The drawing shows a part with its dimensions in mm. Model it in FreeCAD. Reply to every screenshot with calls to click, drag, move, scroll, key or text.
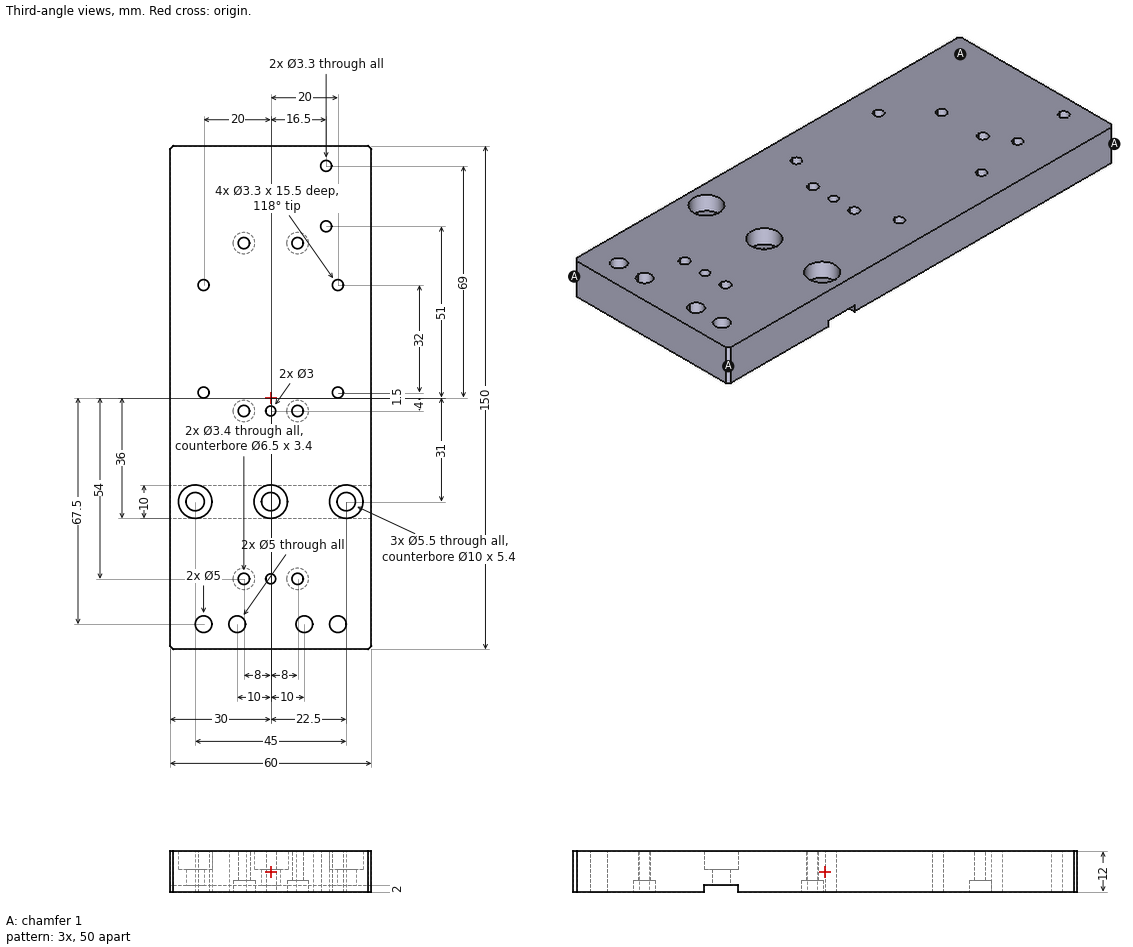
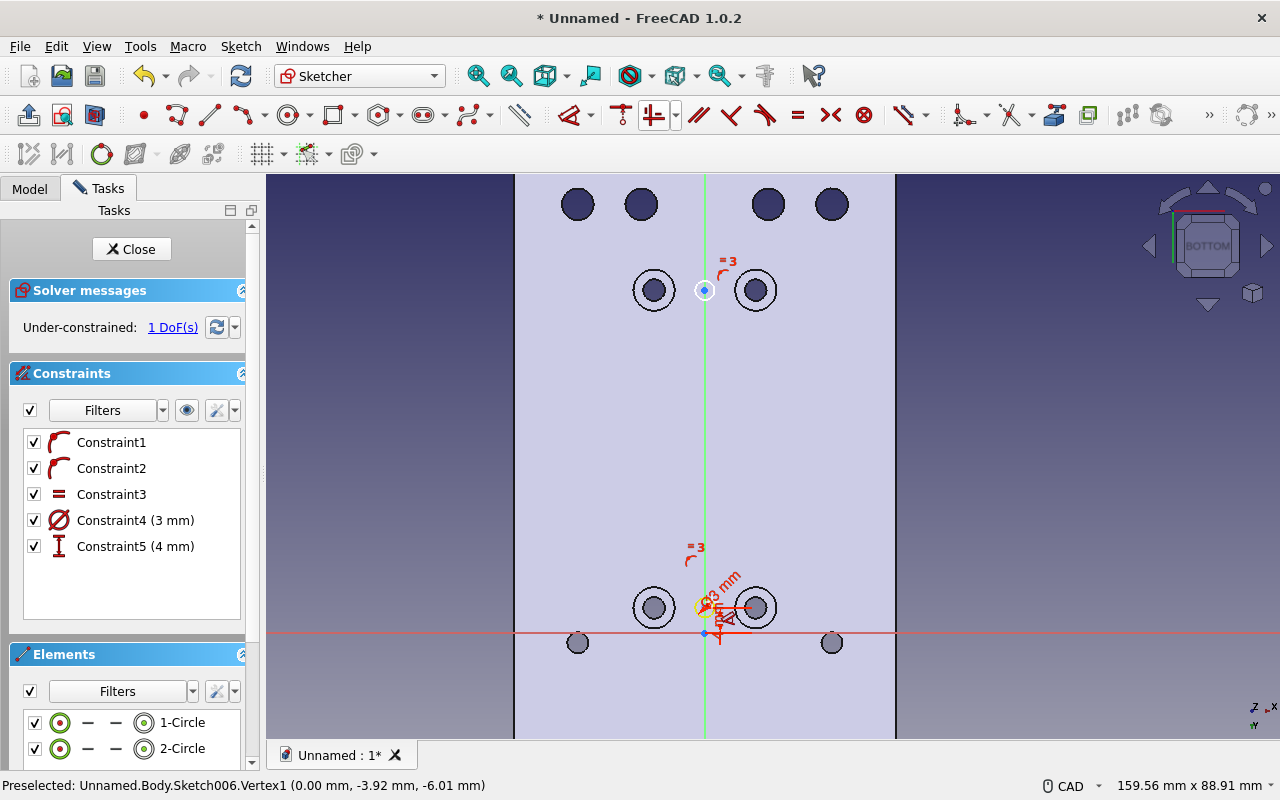
click(705, 290)
click(739, 462)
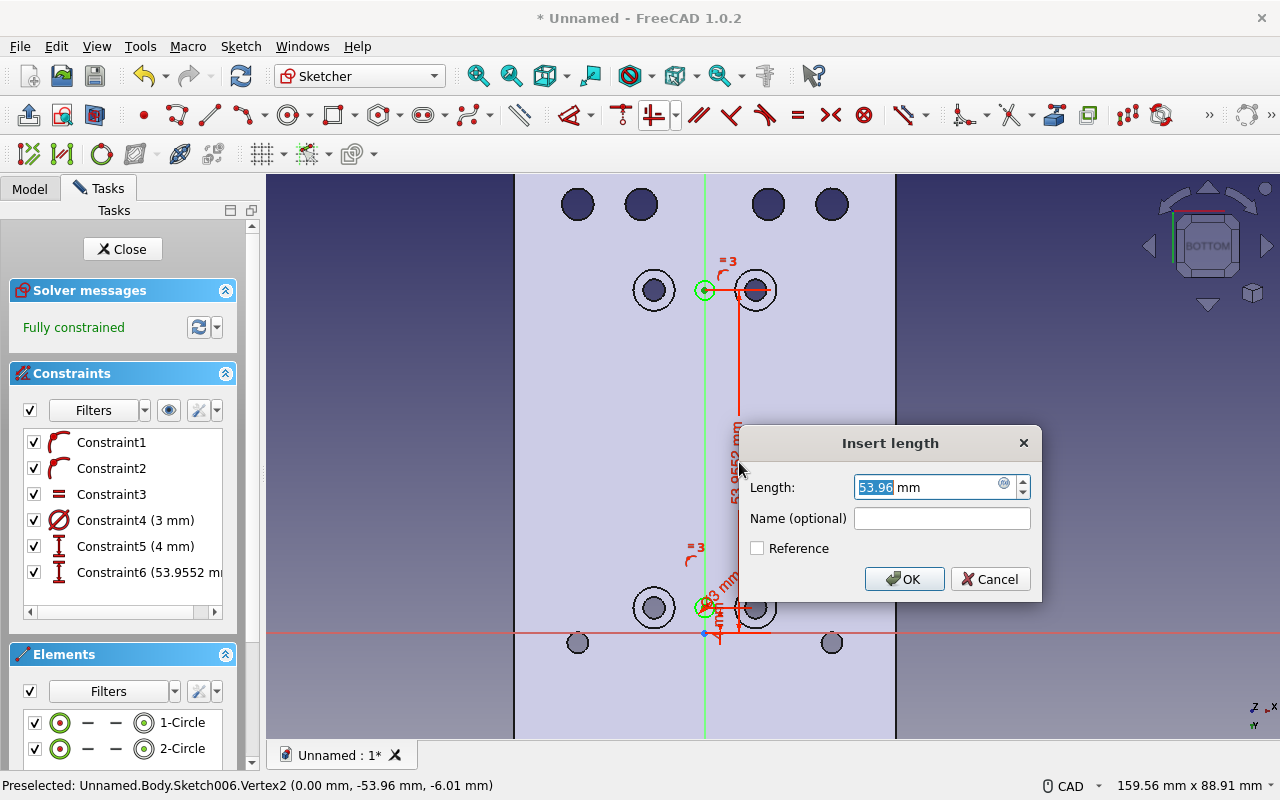
text(54)
key(Return)
key(Escape)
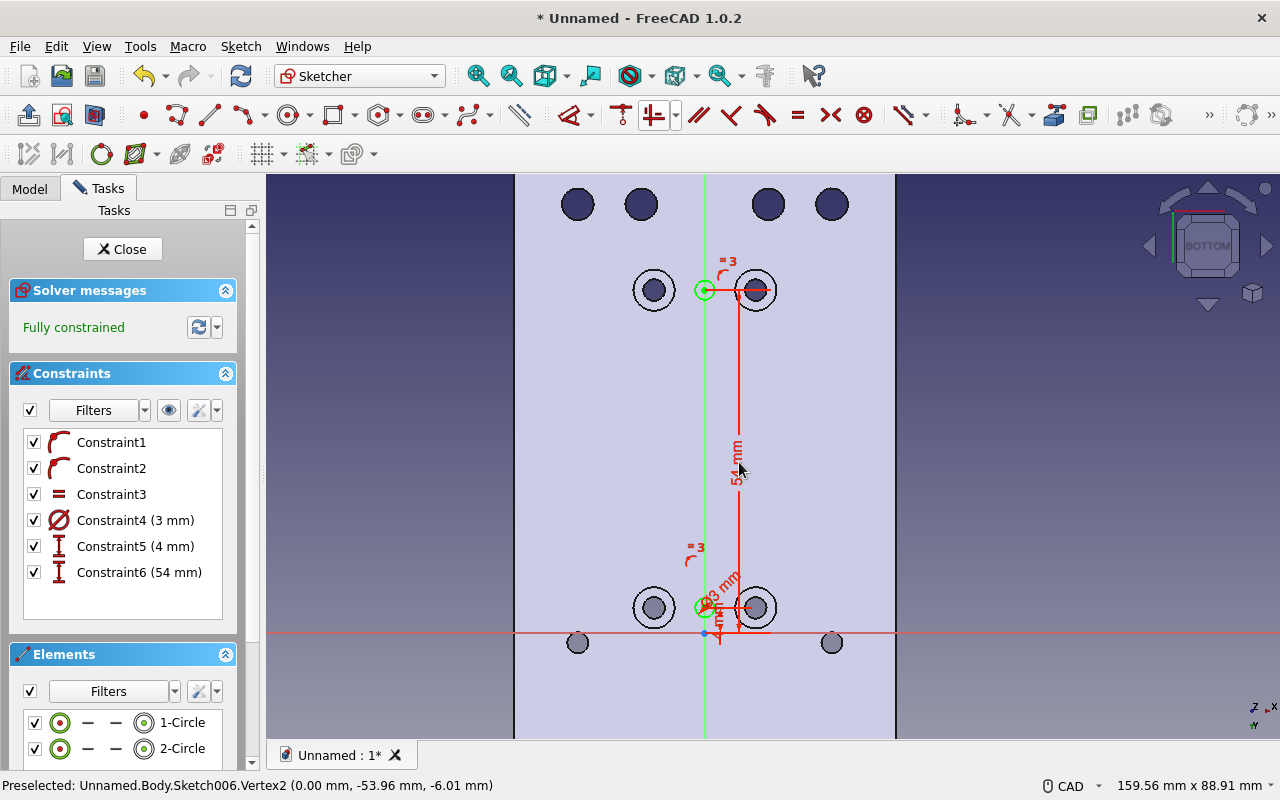
click(123, 249)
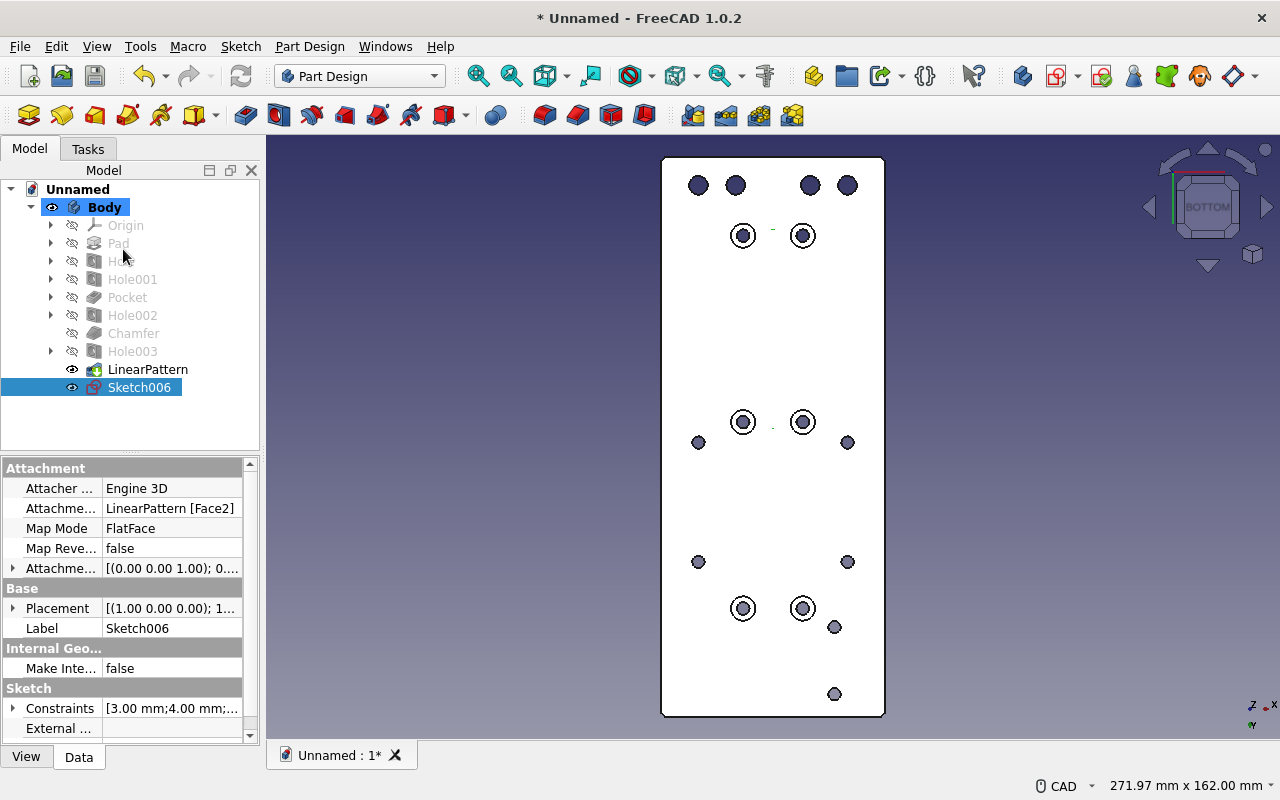
click(246, 116)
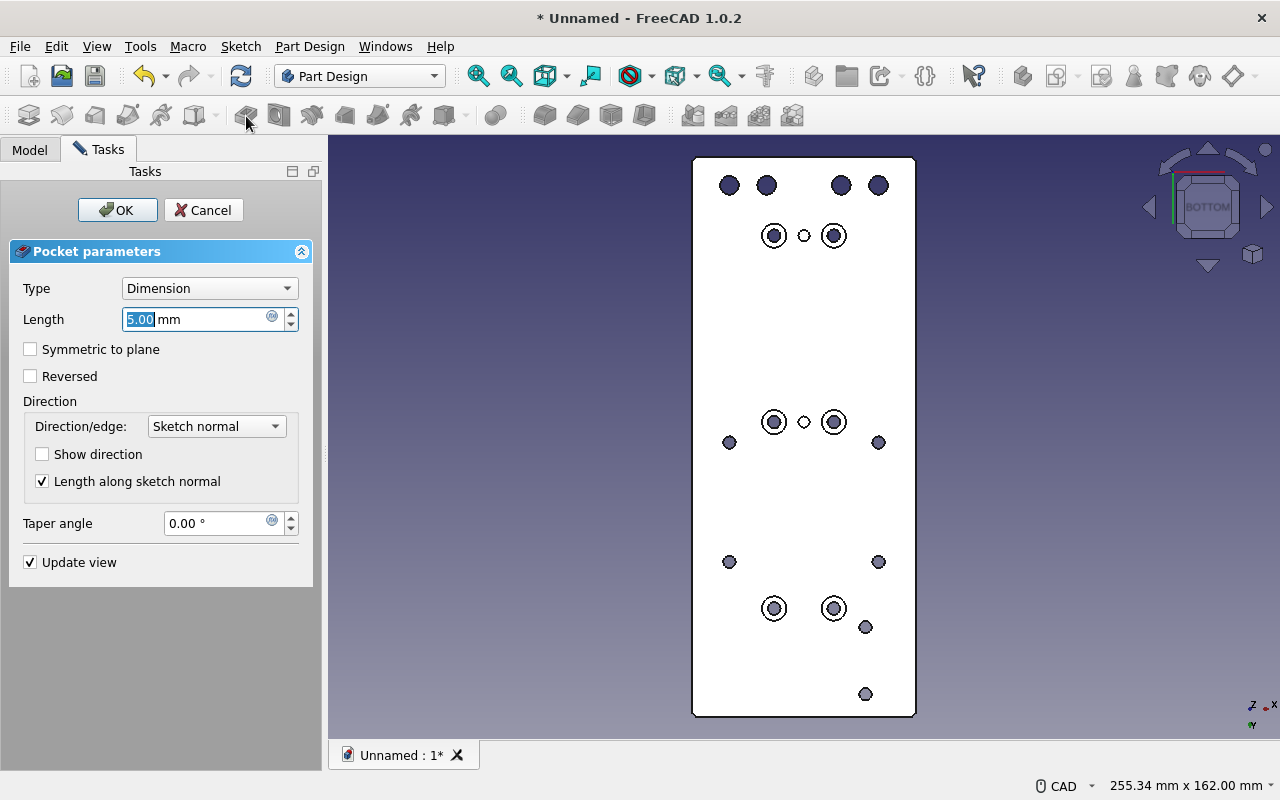
click(210, 288)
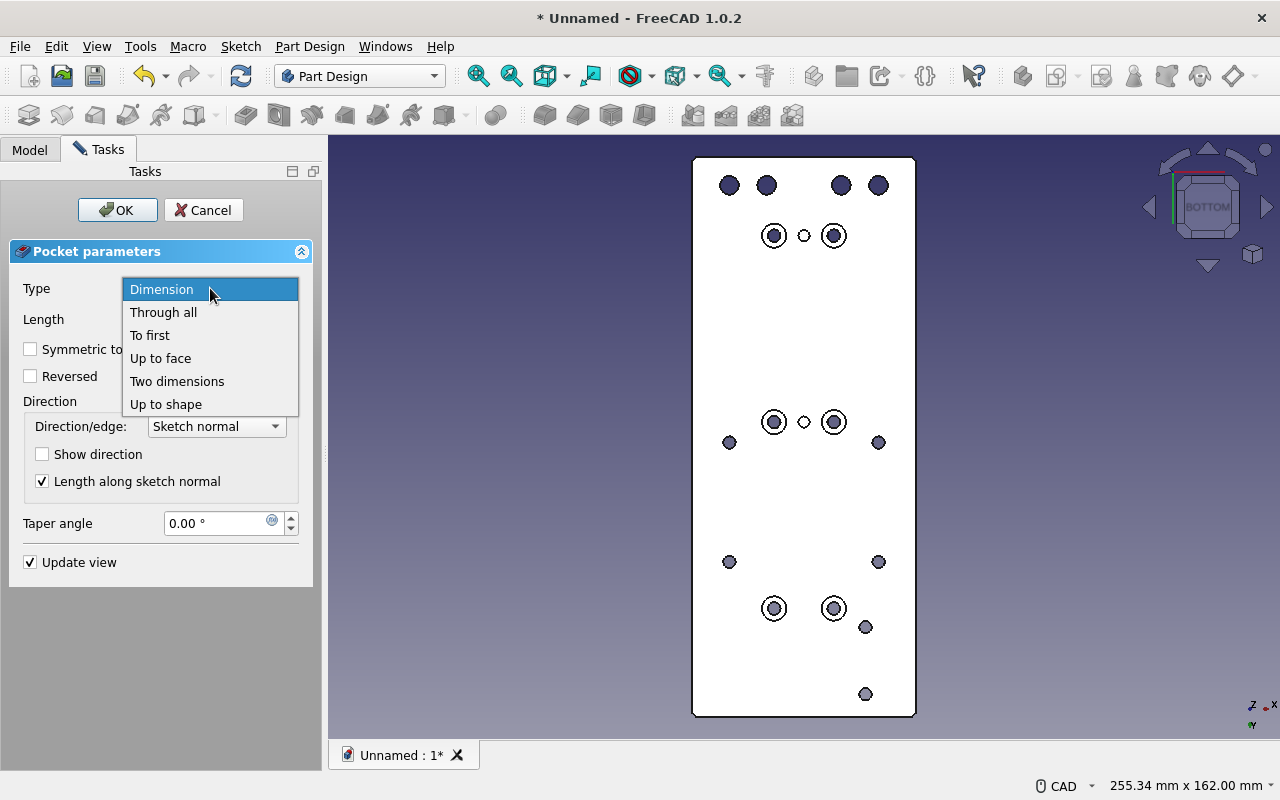
click(208, 312)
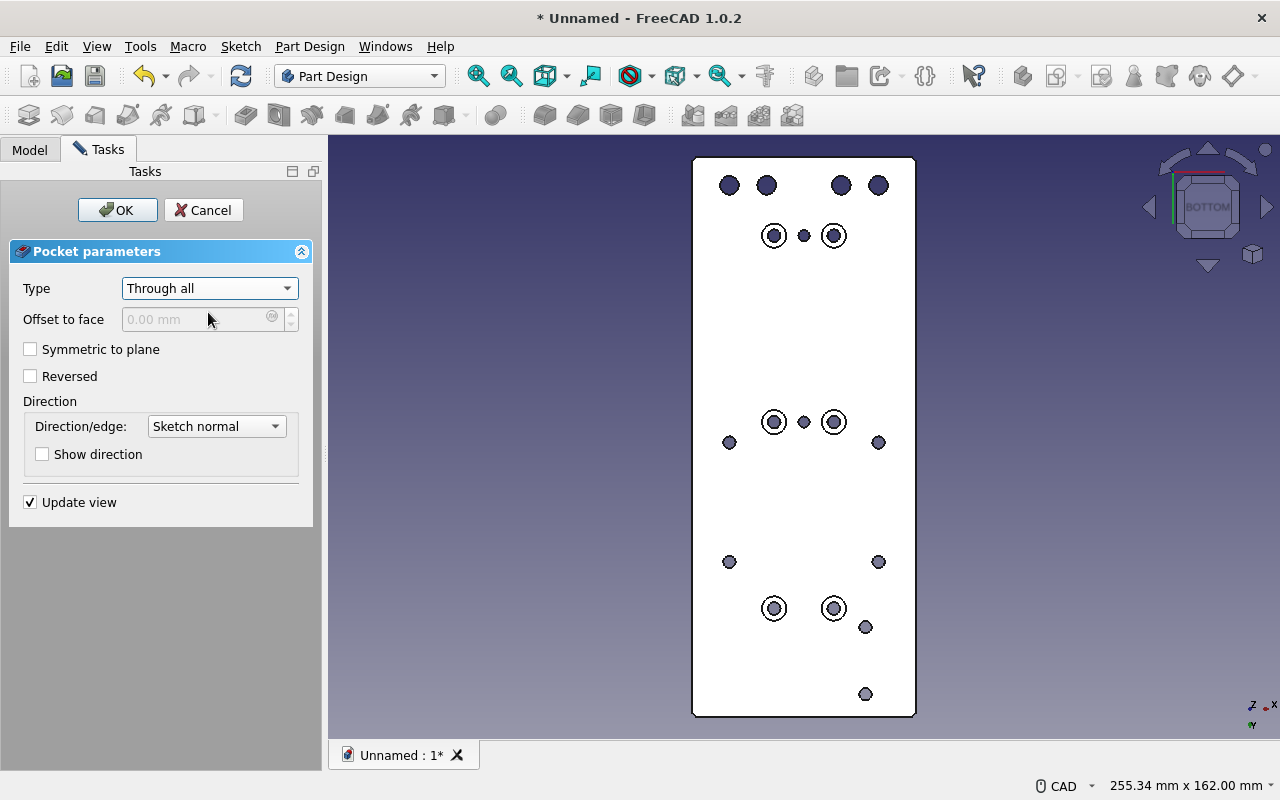
click(118, 210)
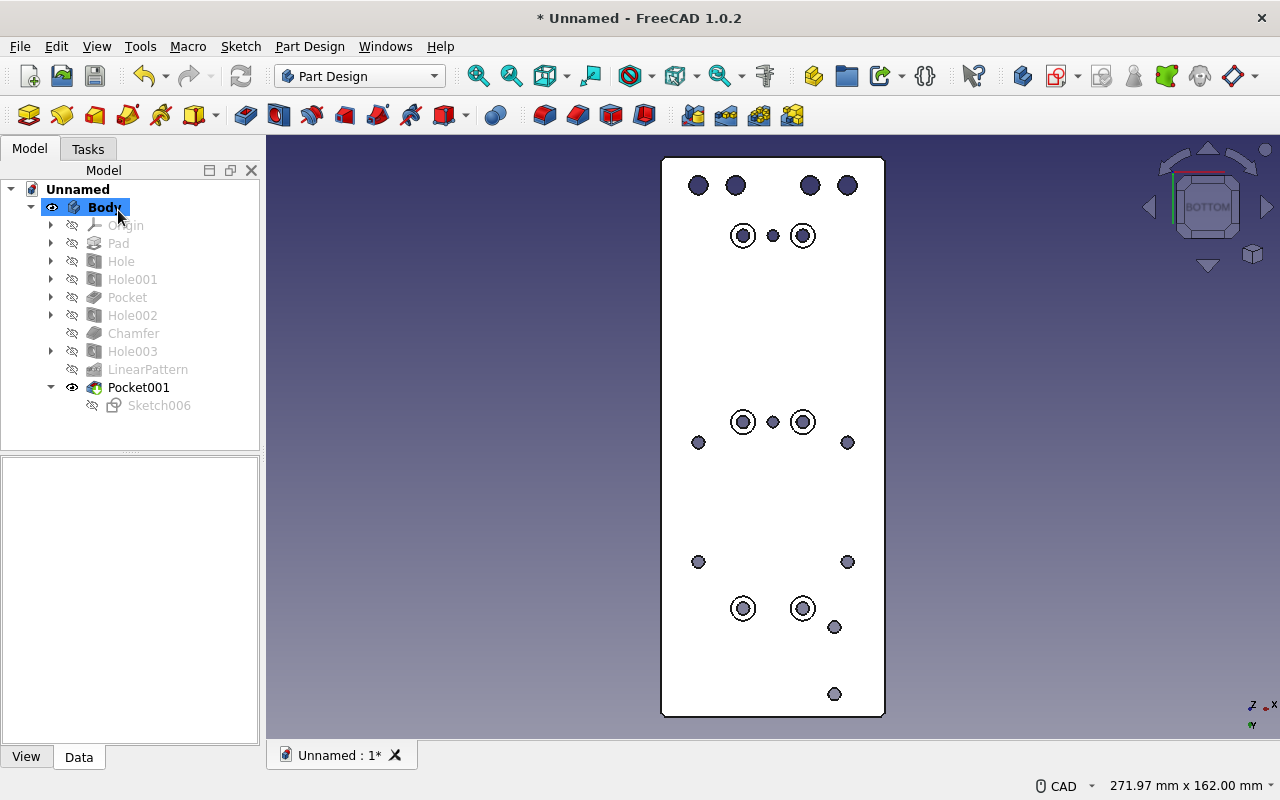
click(773, 516)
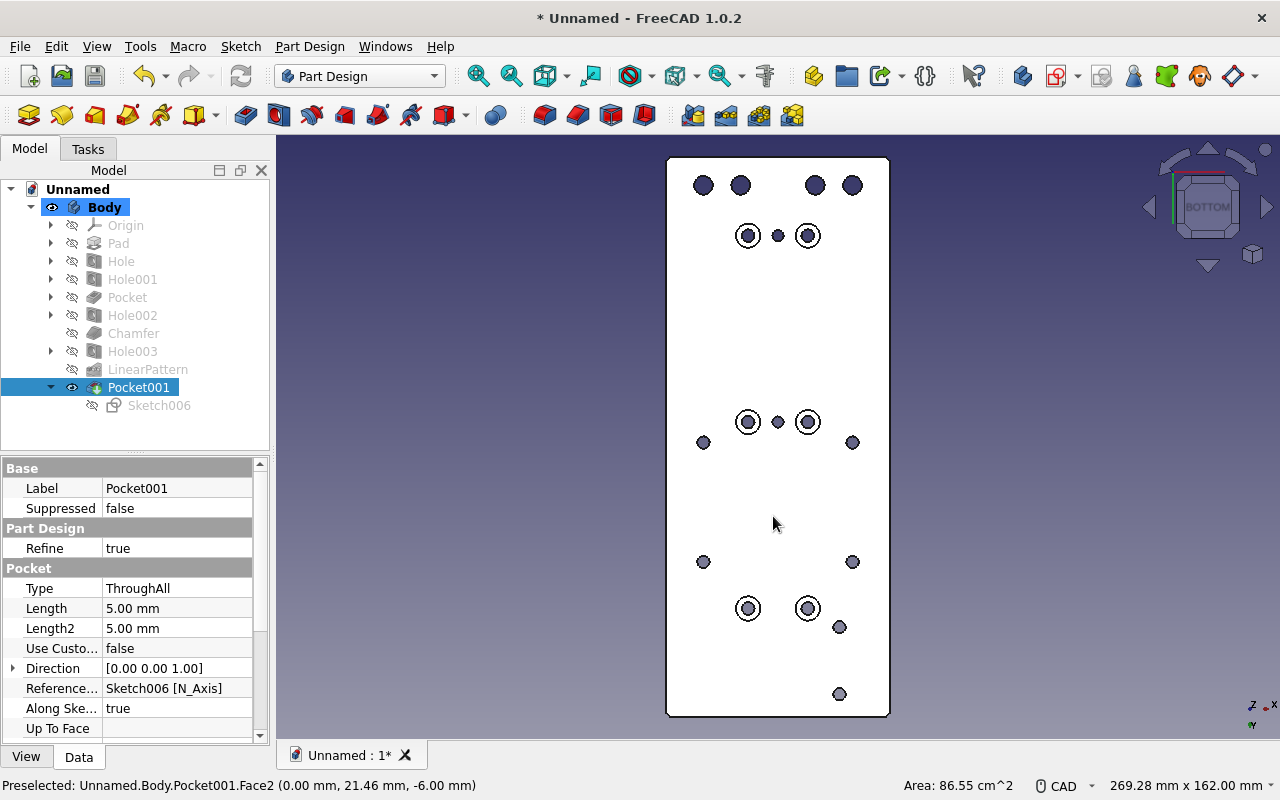
click(1056, 76)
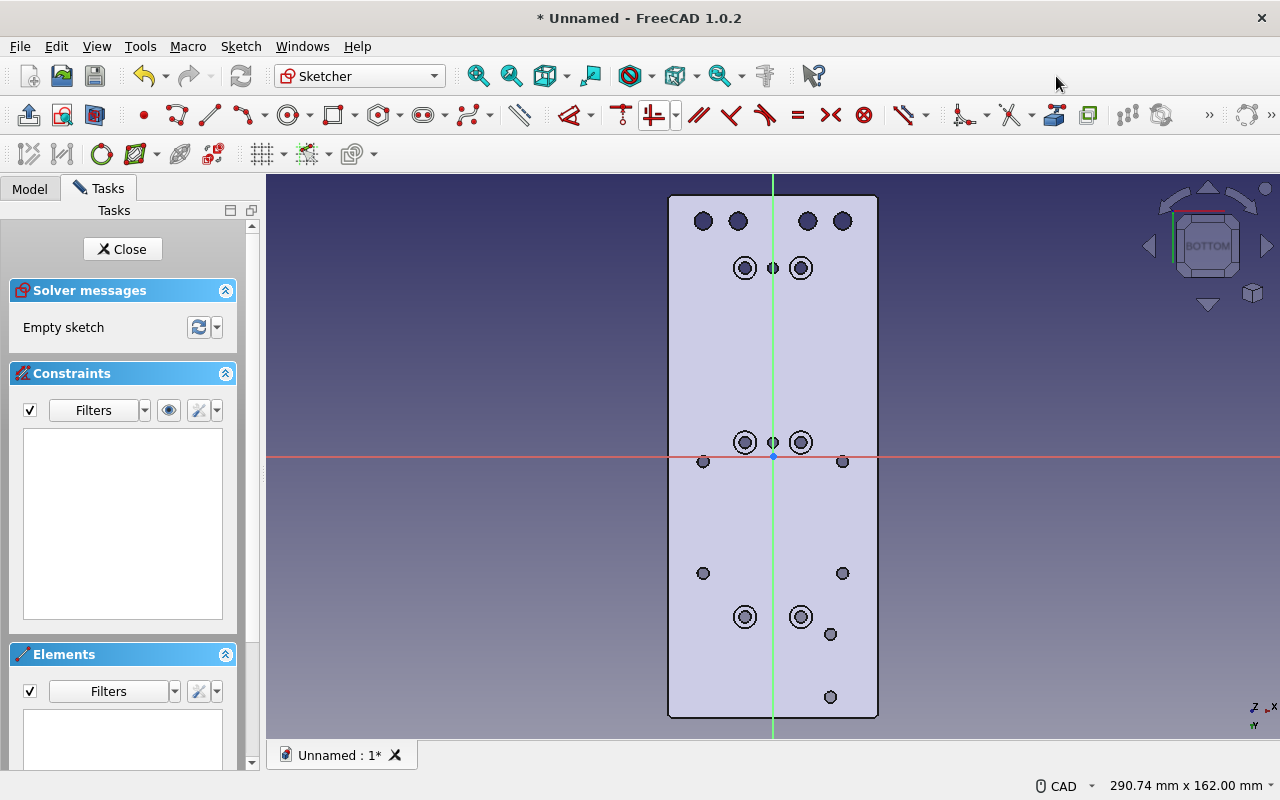
scroll(813, 357, up, 5)